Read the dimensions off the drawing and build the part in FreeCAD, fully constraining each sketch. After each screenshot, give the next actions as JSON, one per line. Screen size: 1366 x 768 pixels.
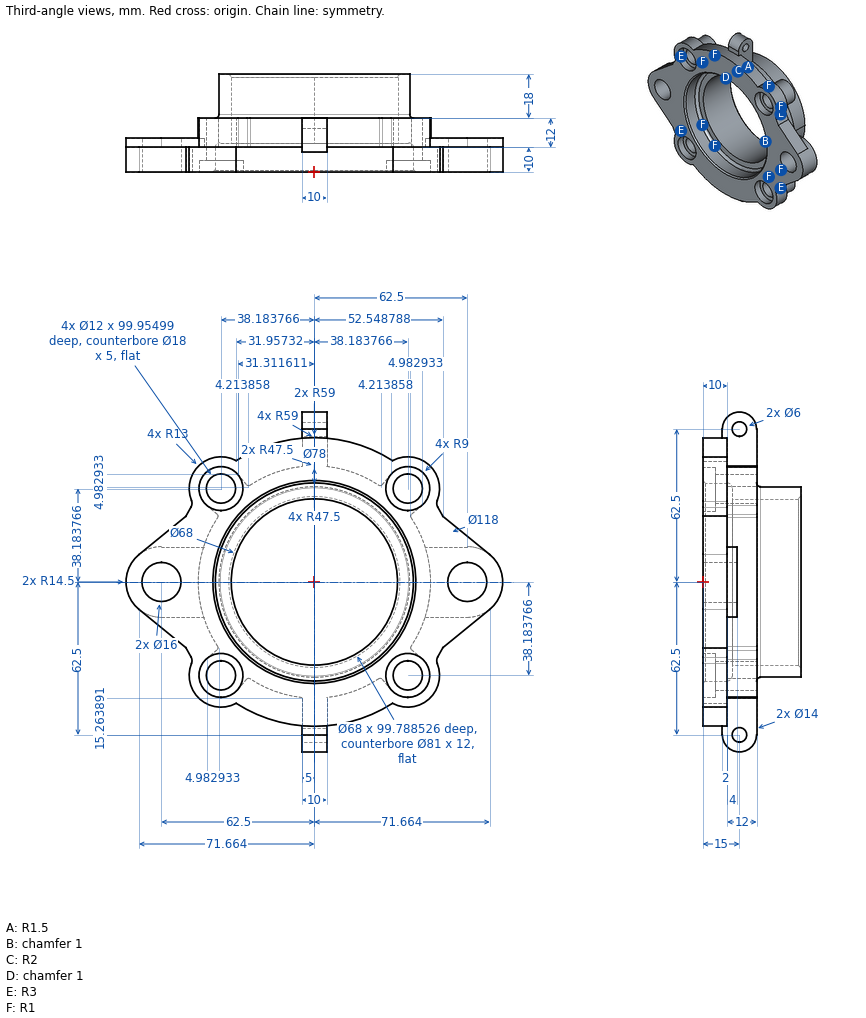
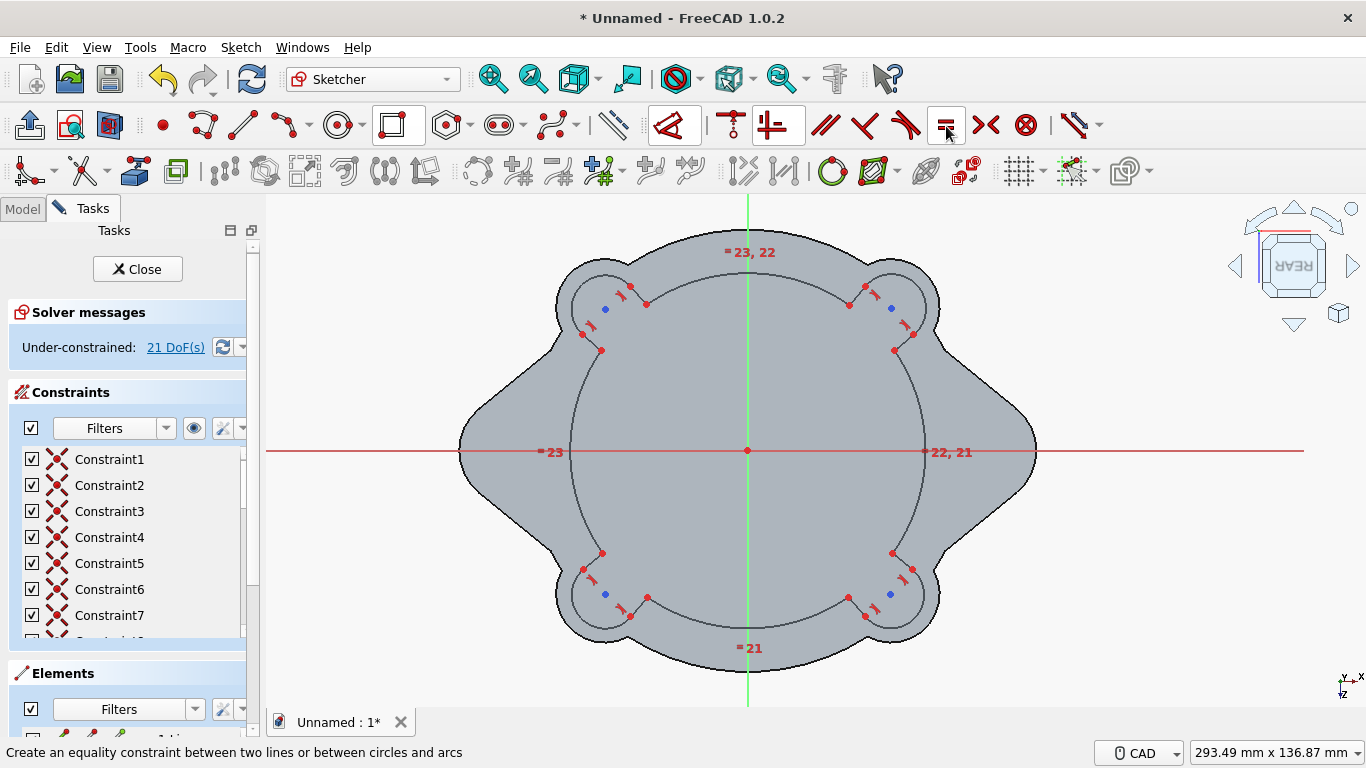
{"action": "left_click", "coordinate": [895, 628]}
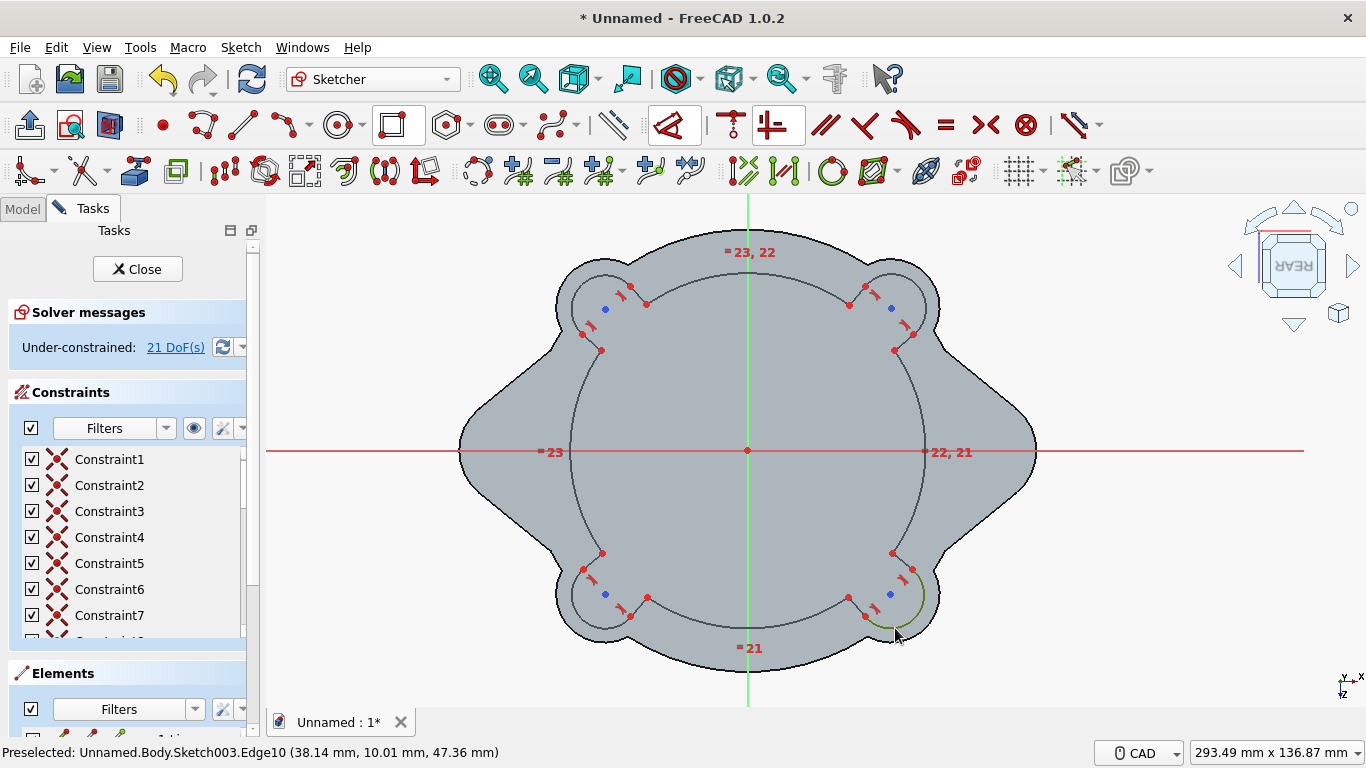
{"action": "left_click", "coordinate": [926, 304]}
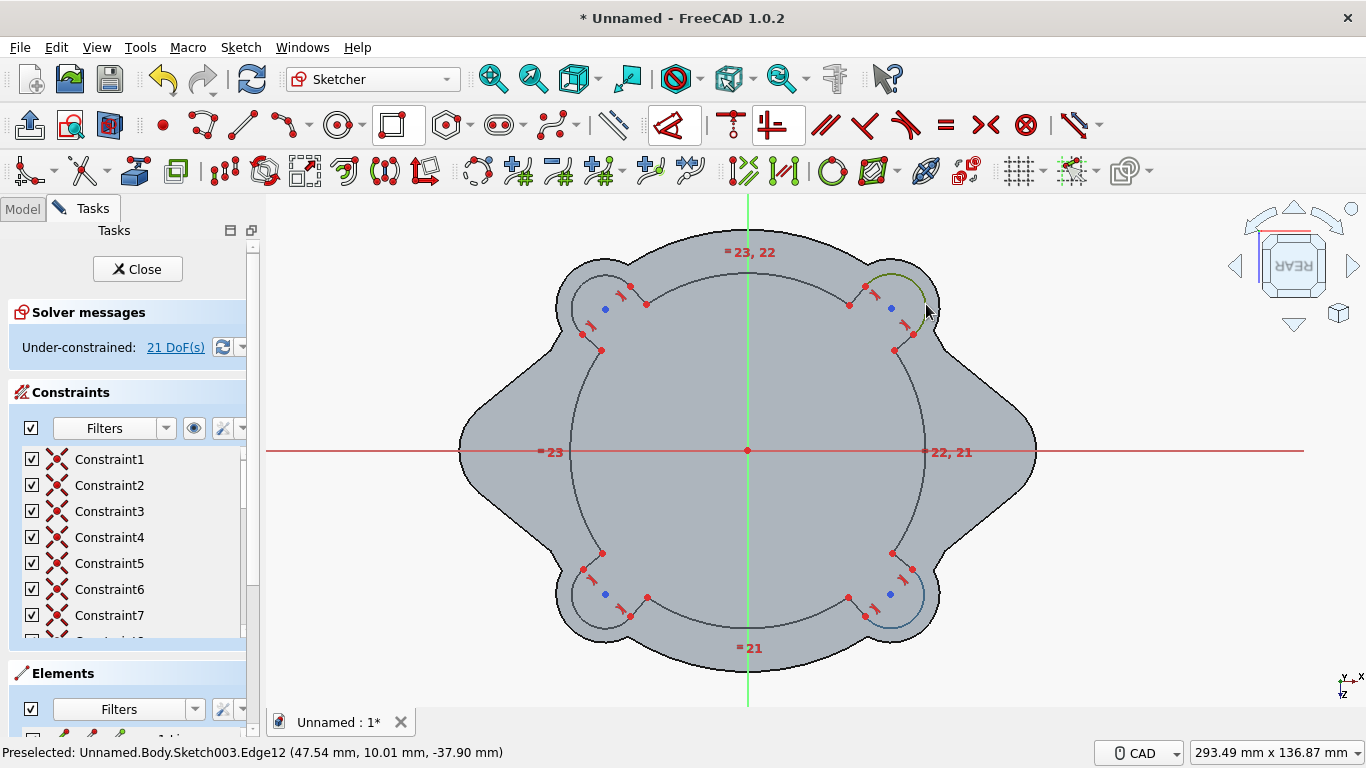
{"action": "left_click", "coordinate": [601, 276]}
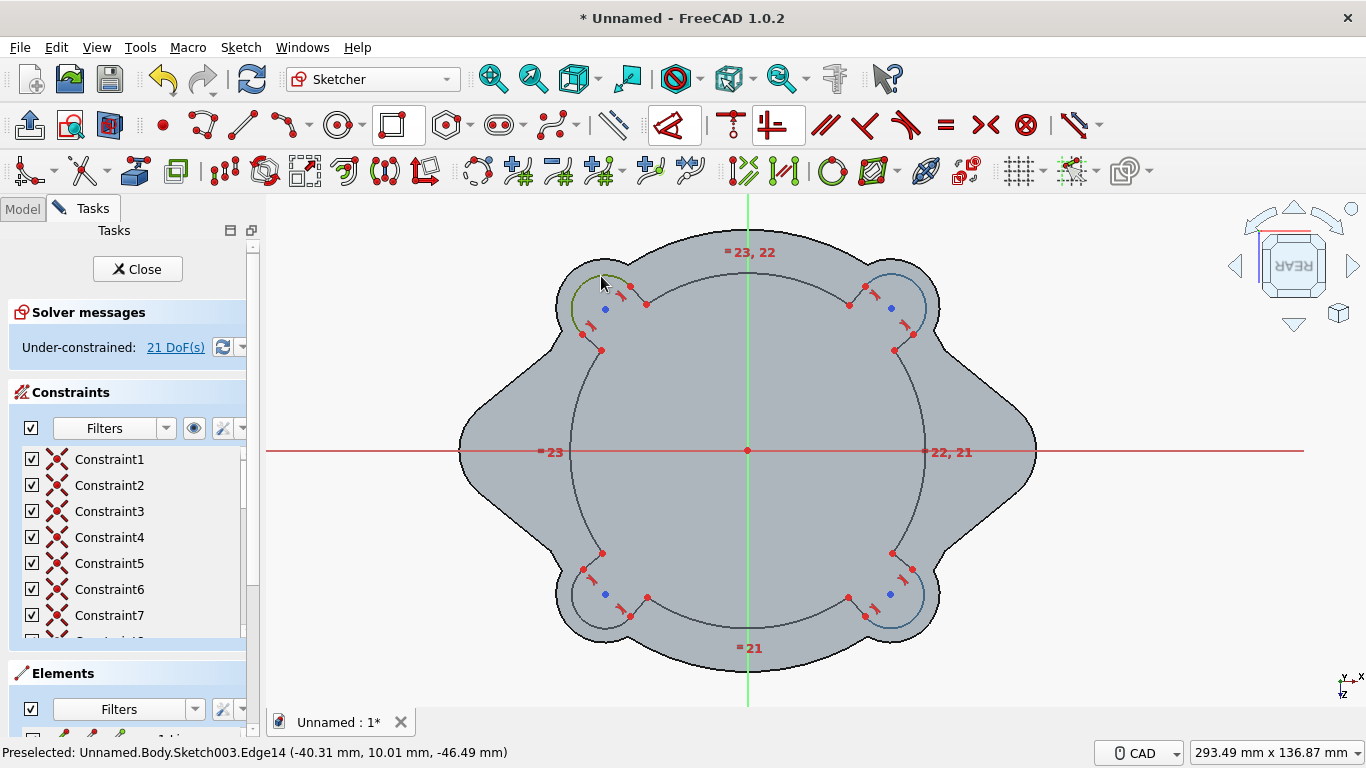
{"action": "left_click", "coordinate": [572, 599]}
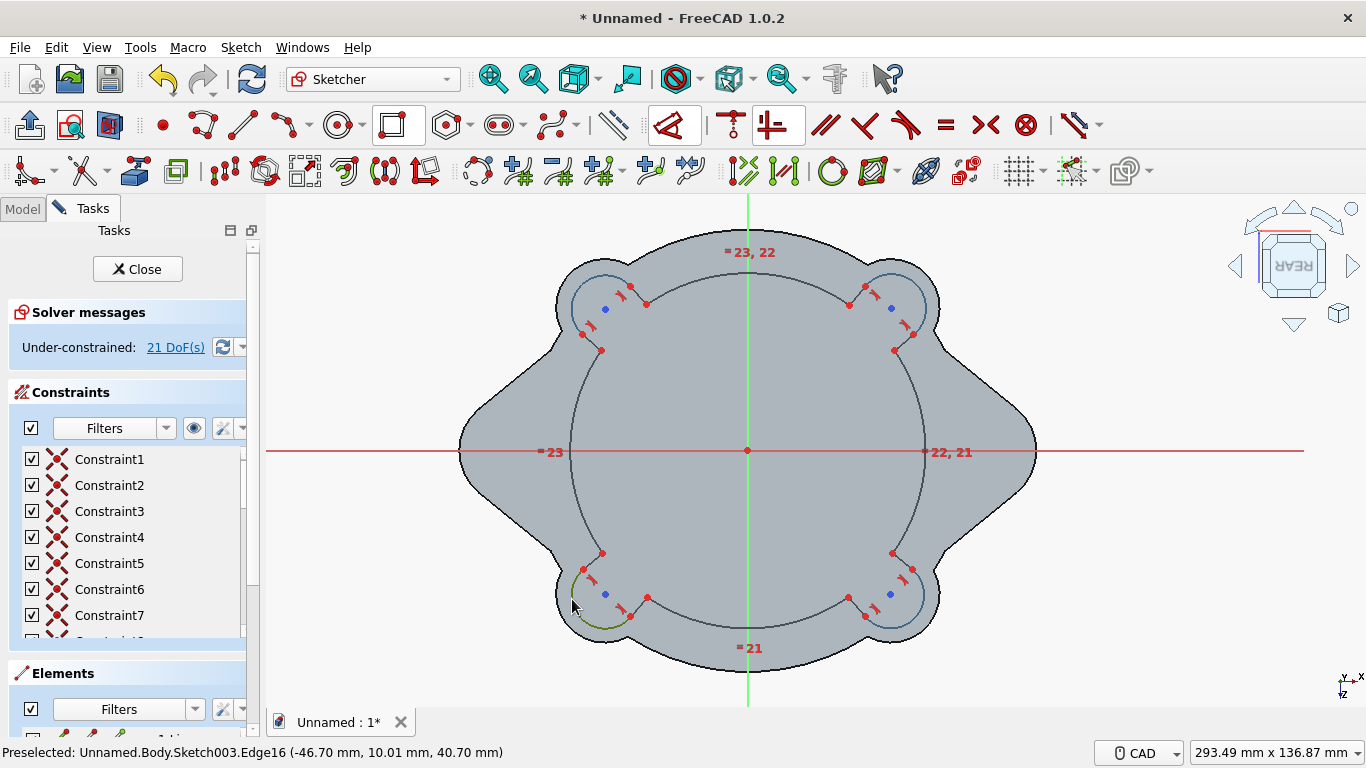
{"action": "left_click", "coordinate": [946, 126]}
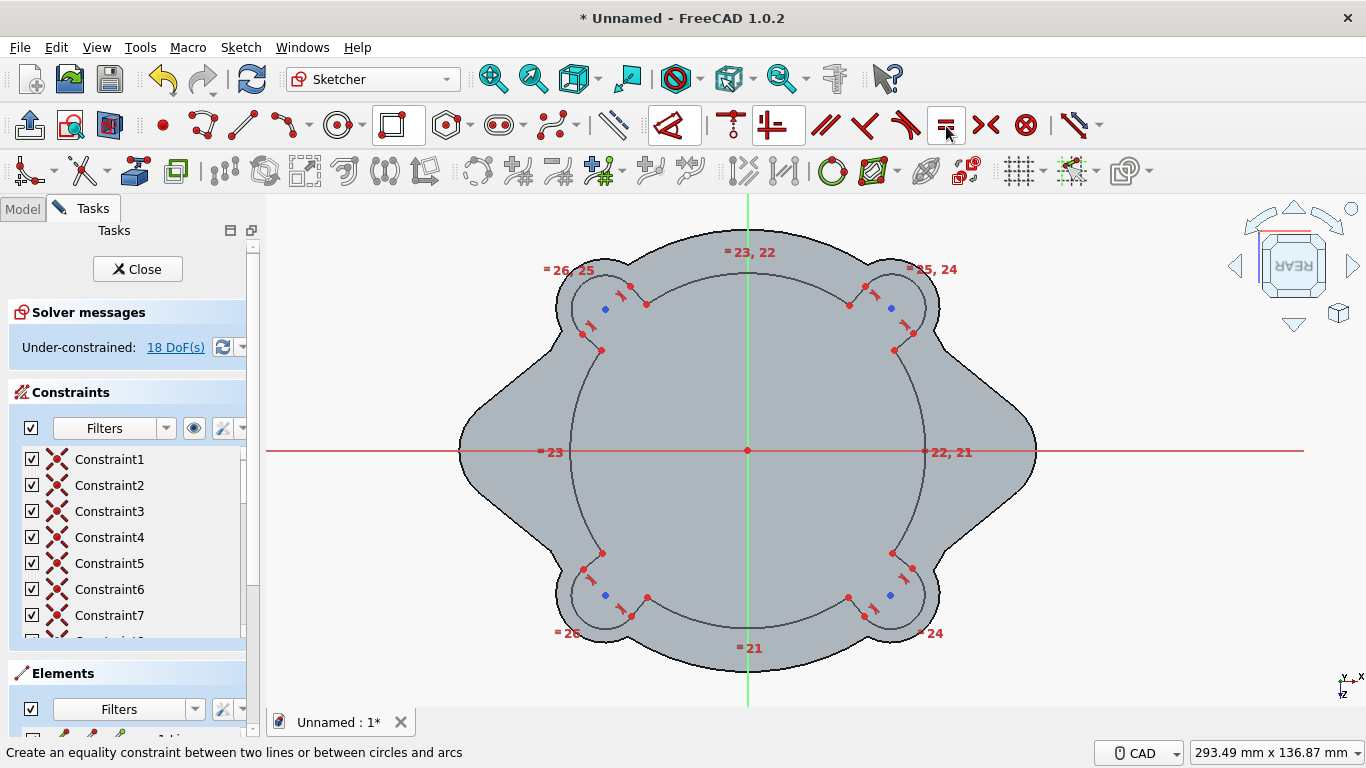
{"action": "left_click", "coordinate": [891, 595]}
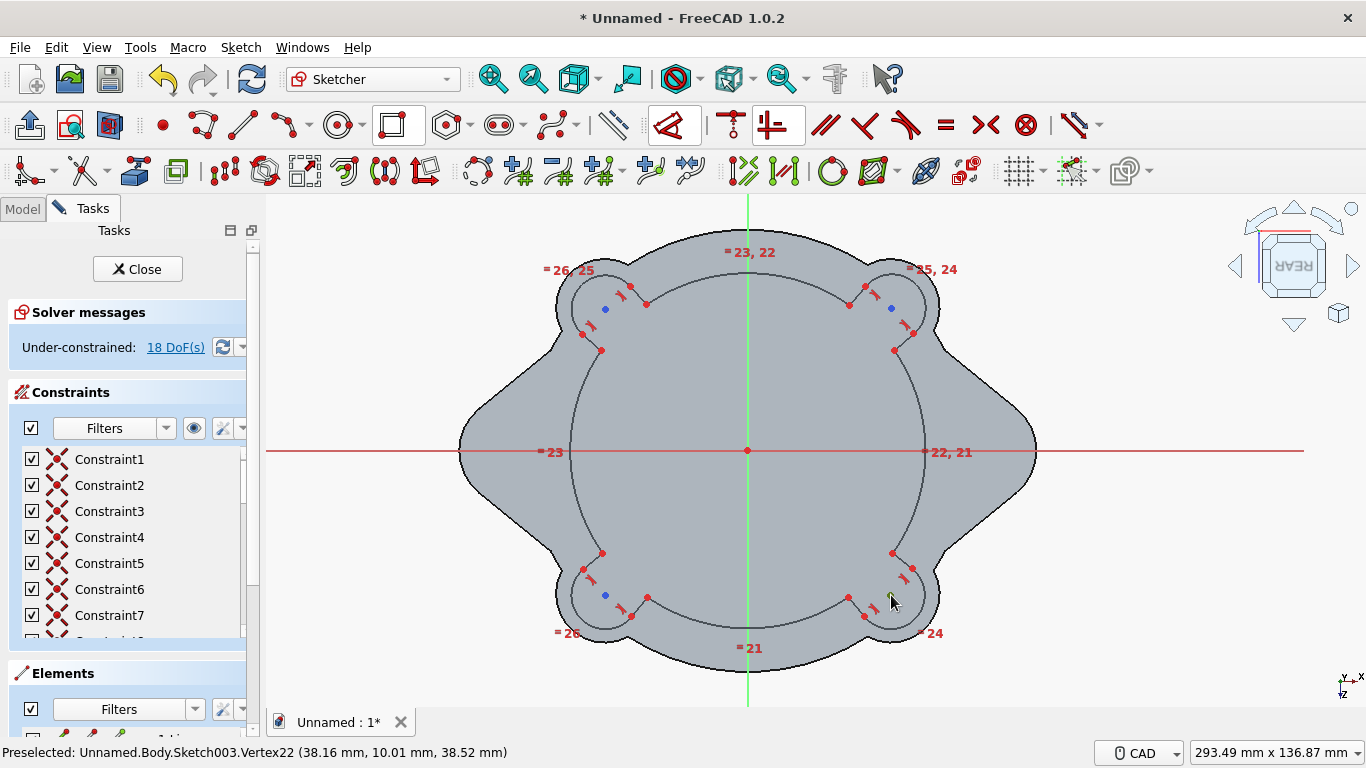
{"action": "left_click", "coordinate": [892, 308]}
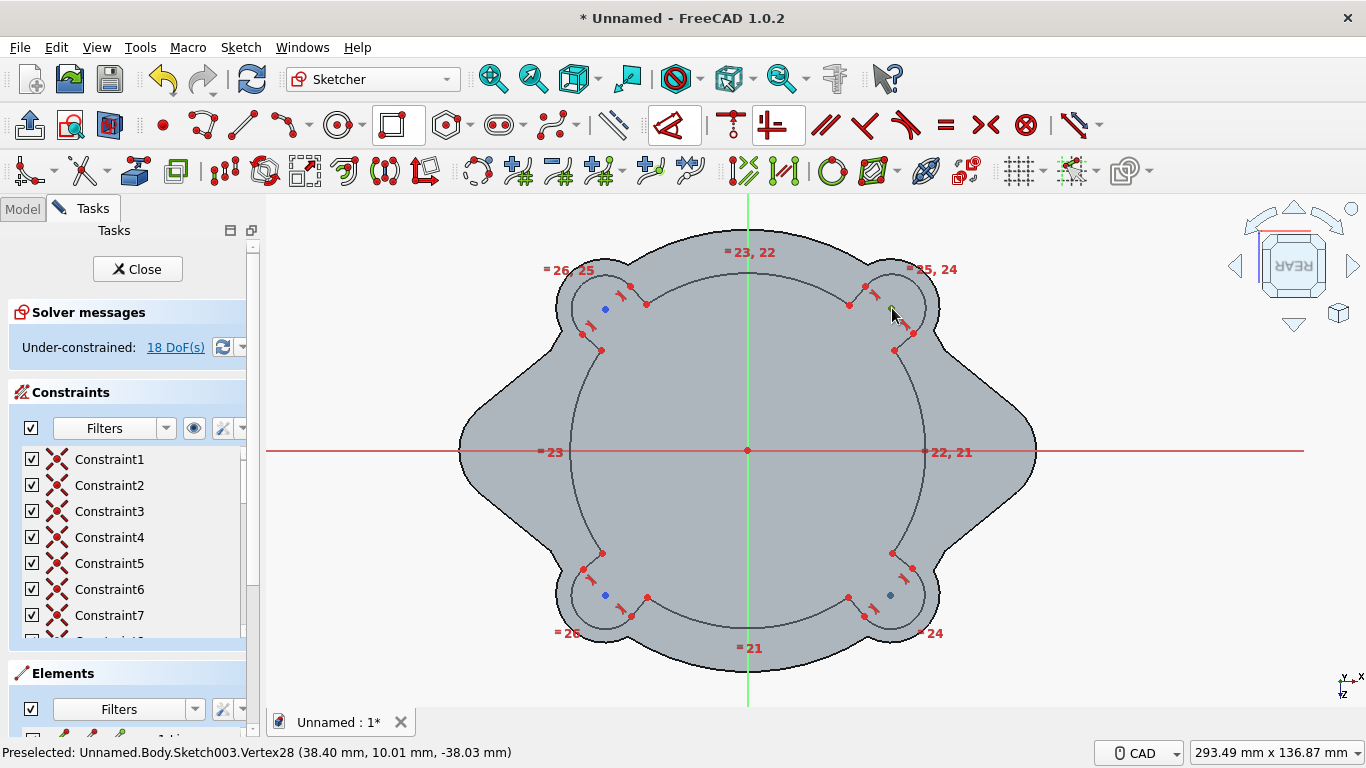
{"action": "left_click", "coordinate": [359, 451]}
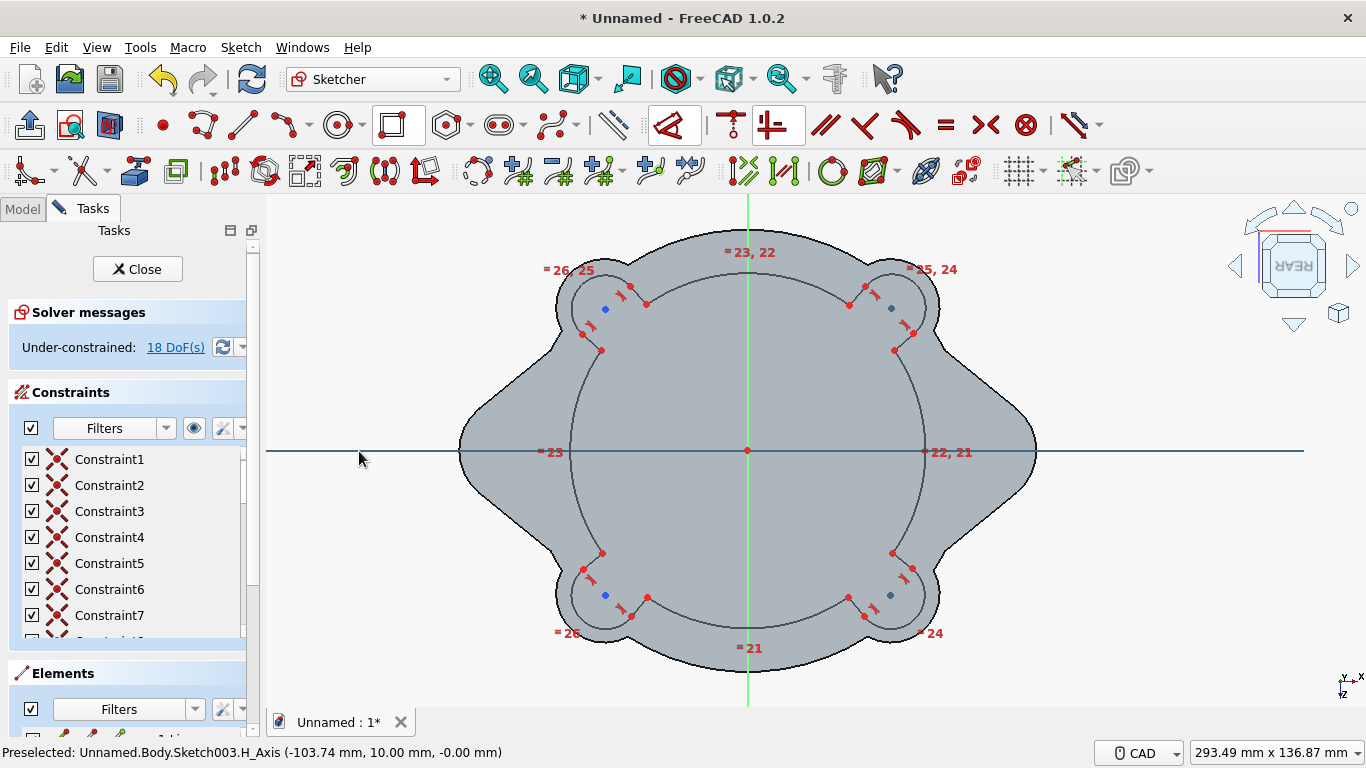
{"action": "left_click", "coordinate": [986, 126]}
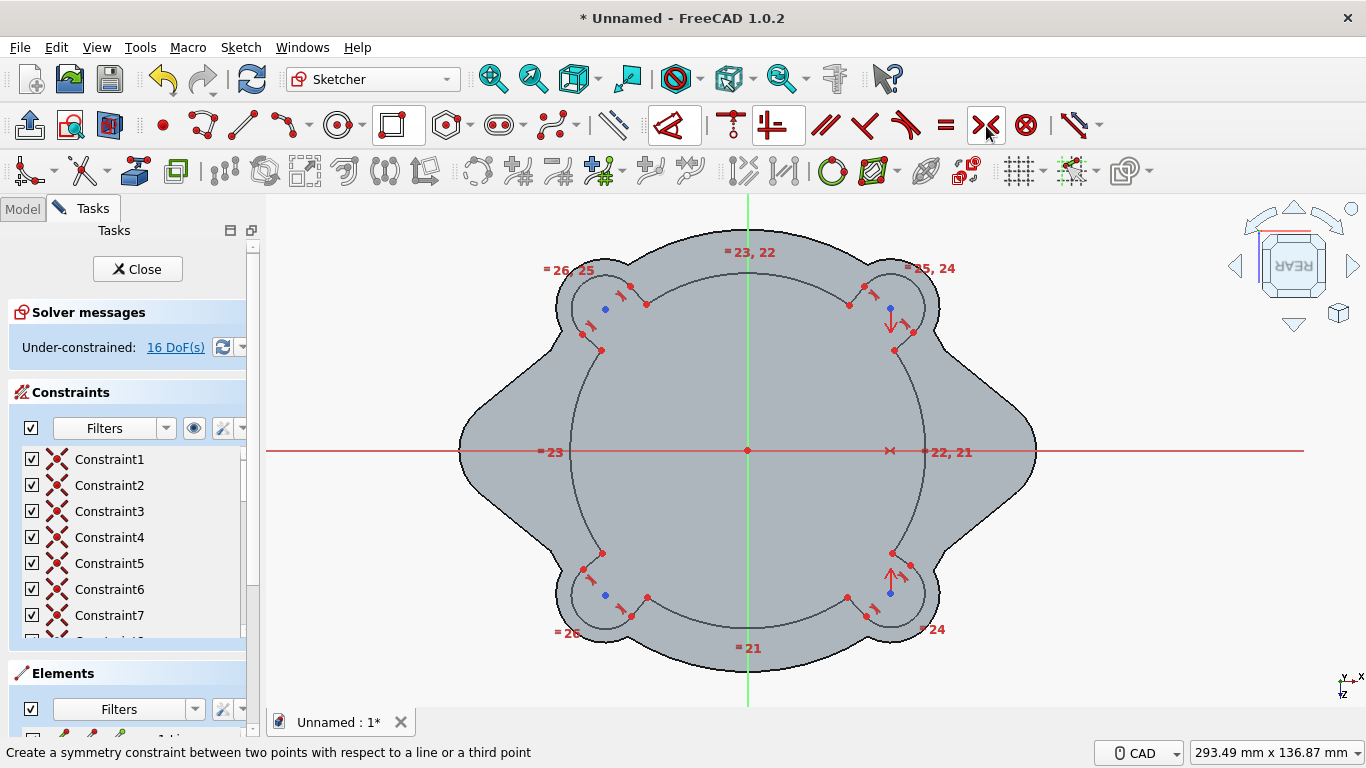
{"action": "left_click", "coordinate": [891, 308]}